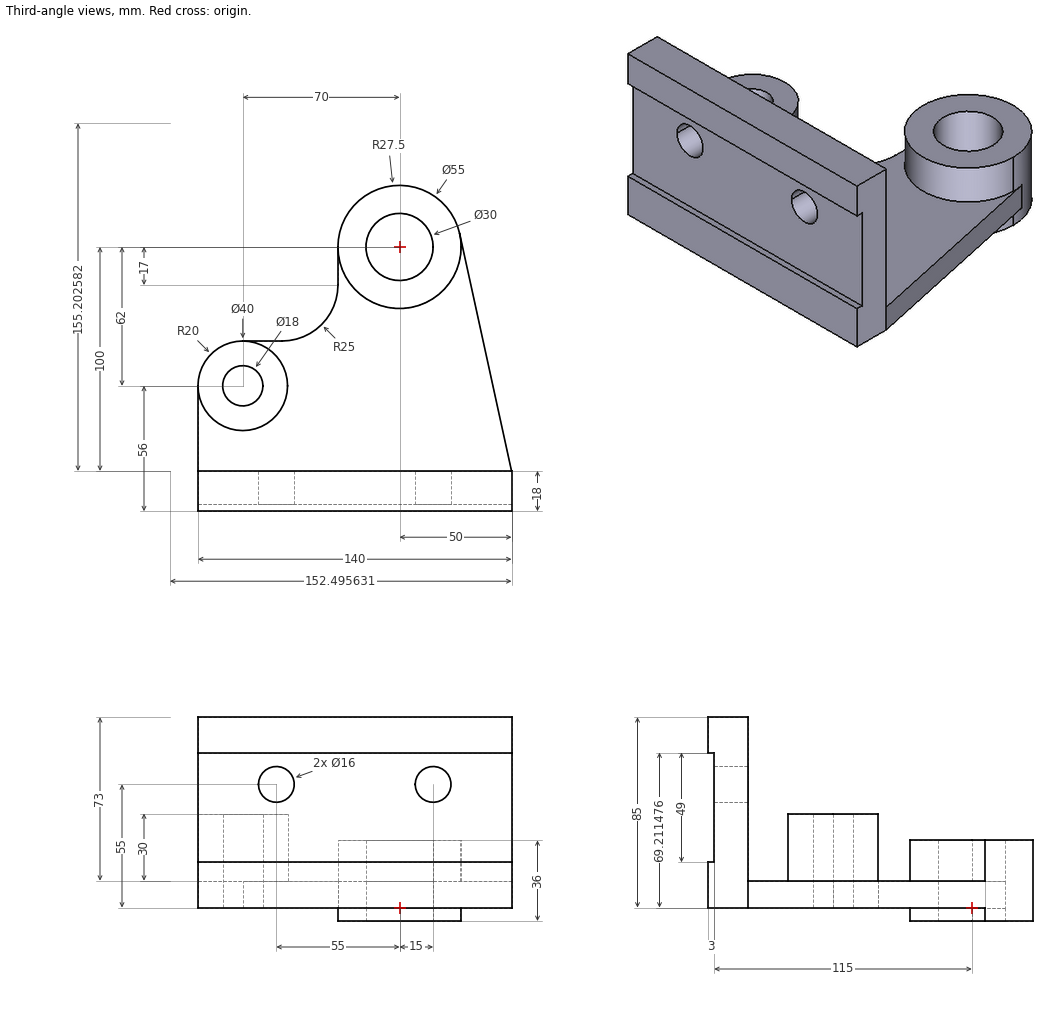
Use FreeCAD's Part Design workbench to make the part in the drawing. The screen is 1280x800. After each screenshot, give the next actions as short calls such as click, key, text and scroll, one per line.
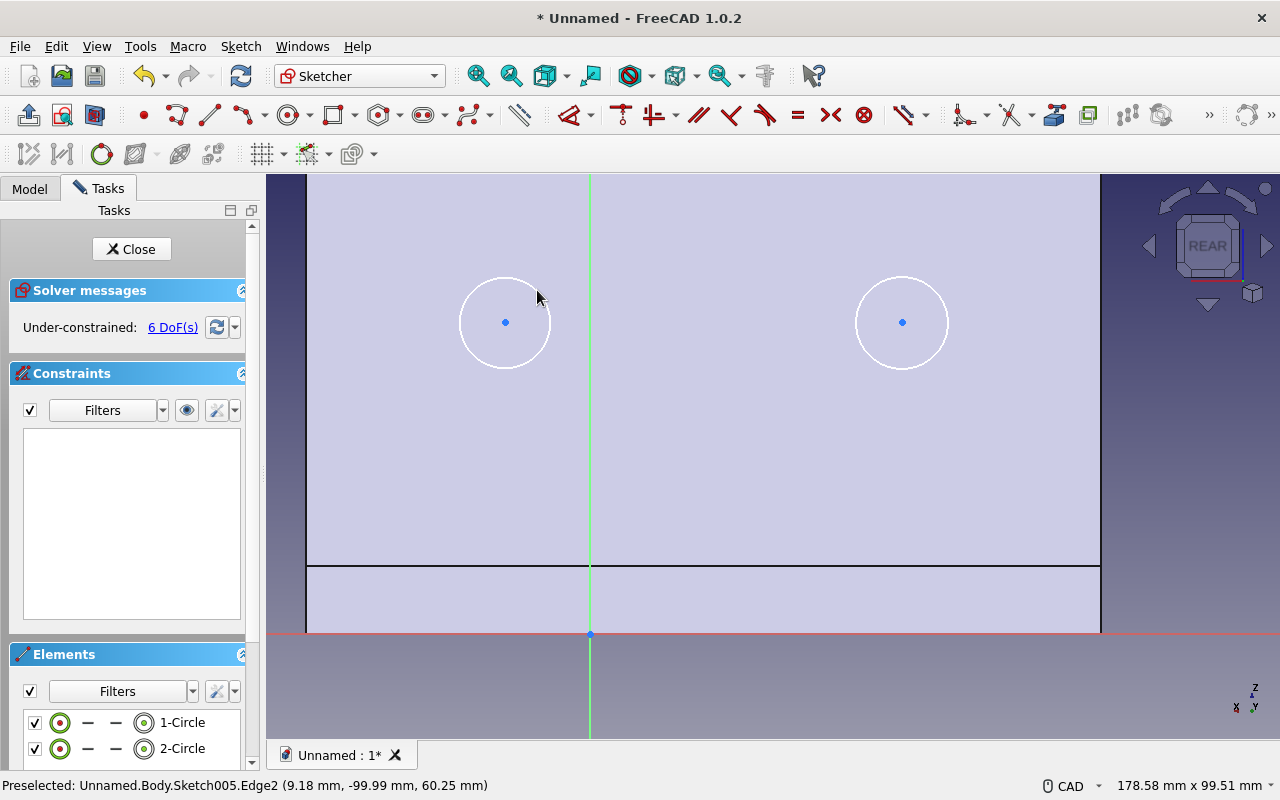
click(934, 290)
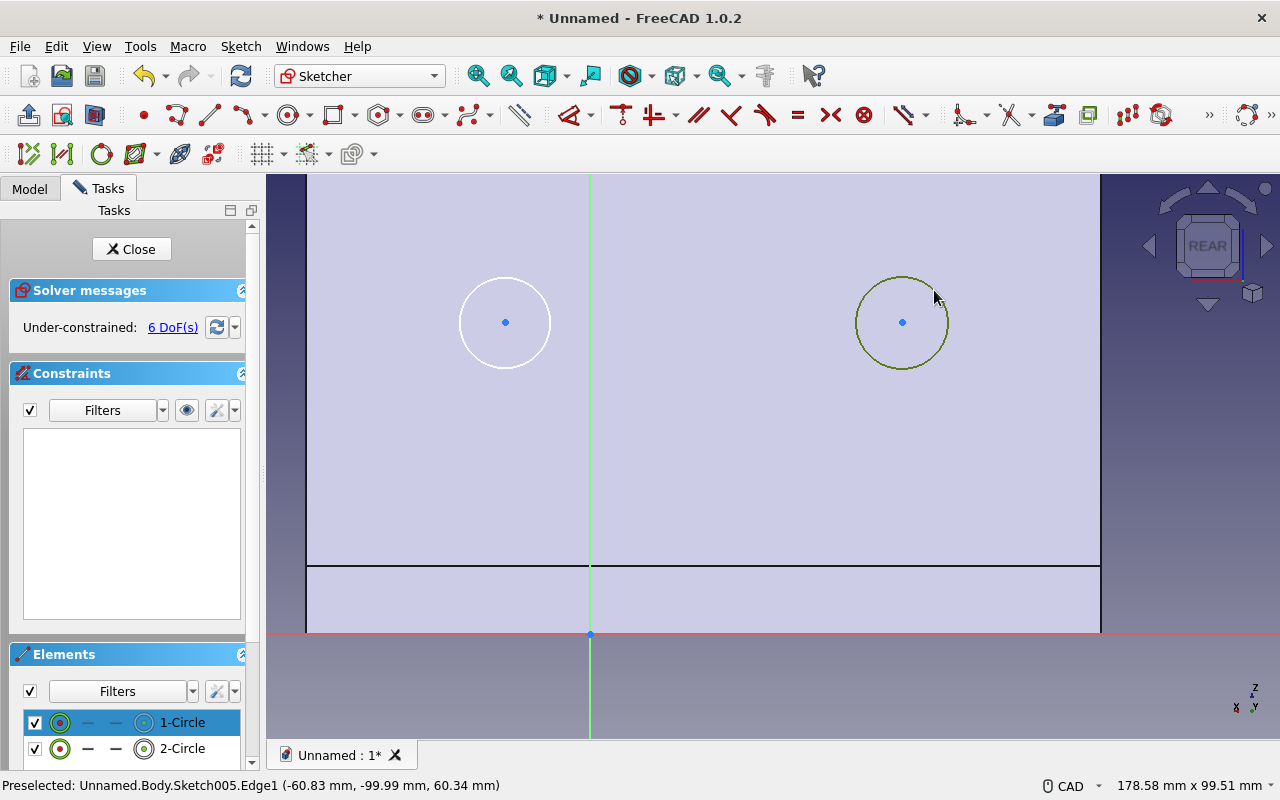
click(537, 291)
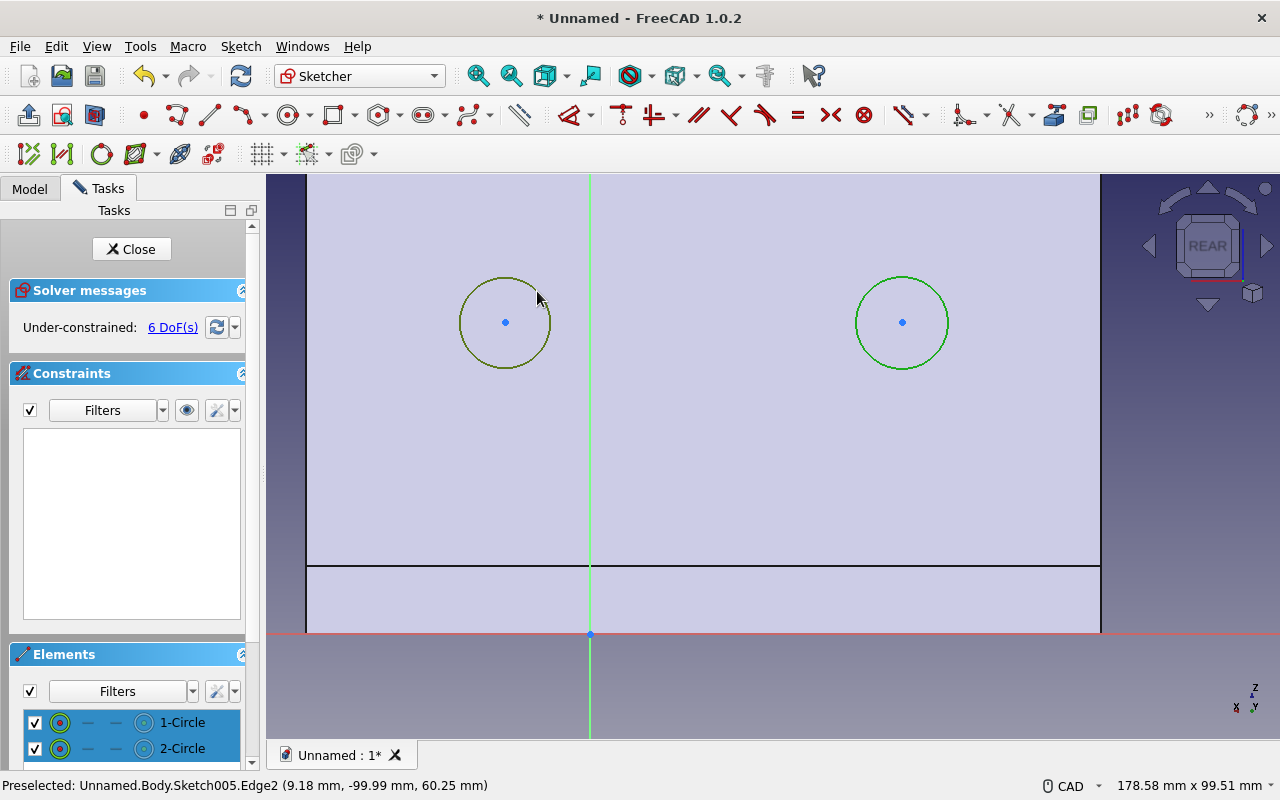
click(798, 116)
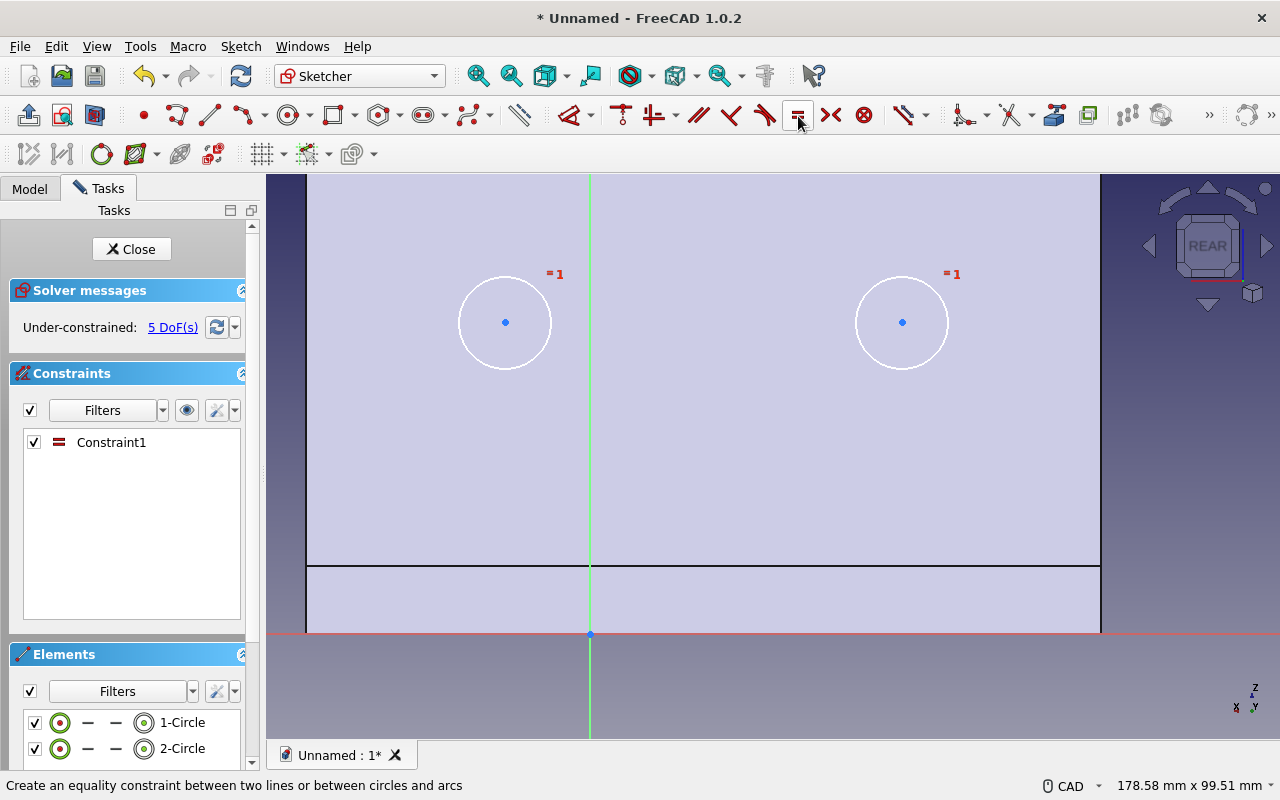
click(902, 323)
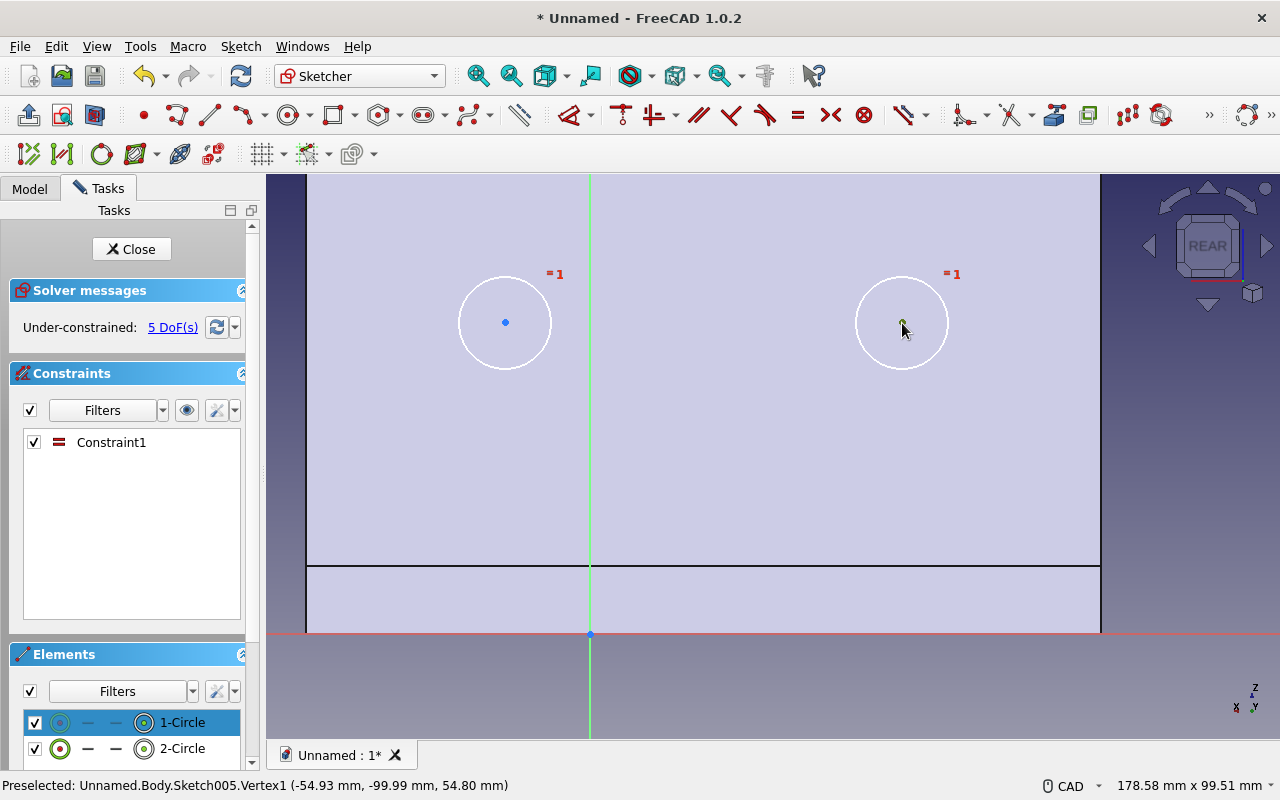
click(505, 323)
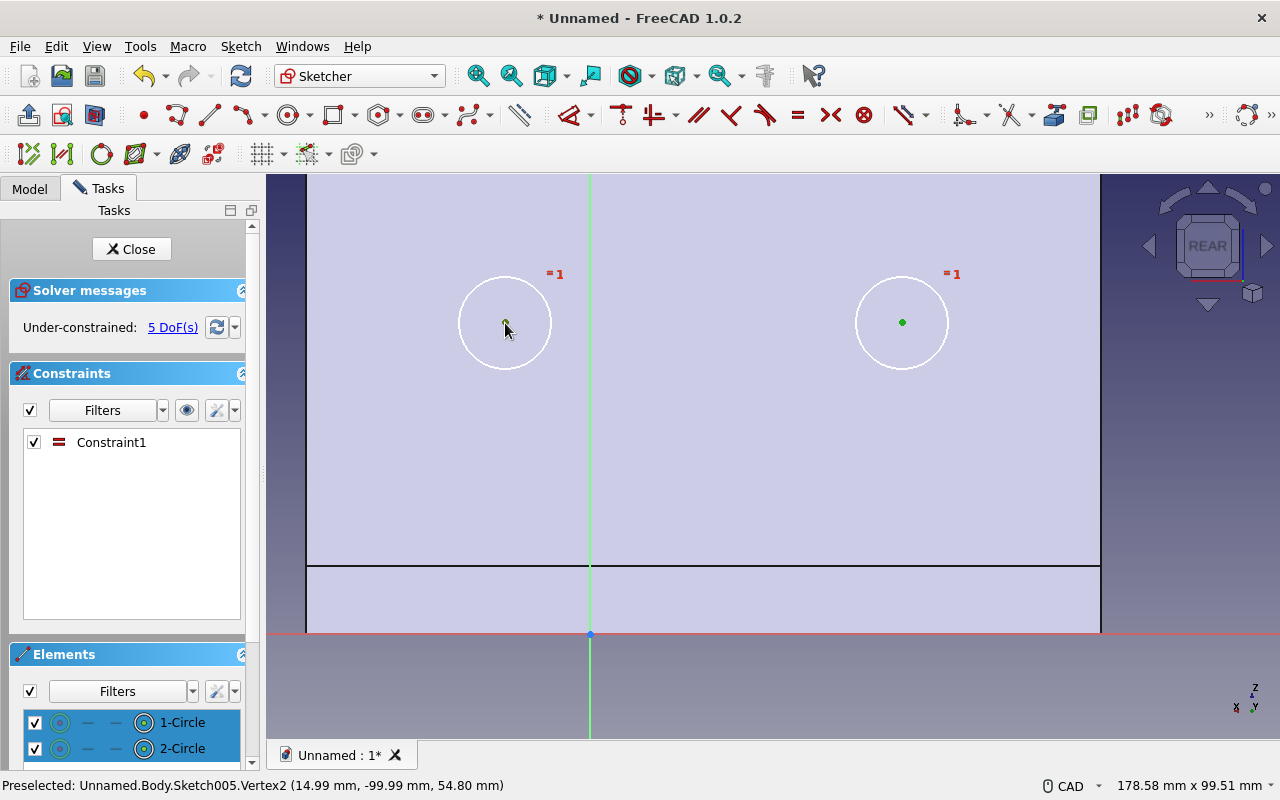
key(h)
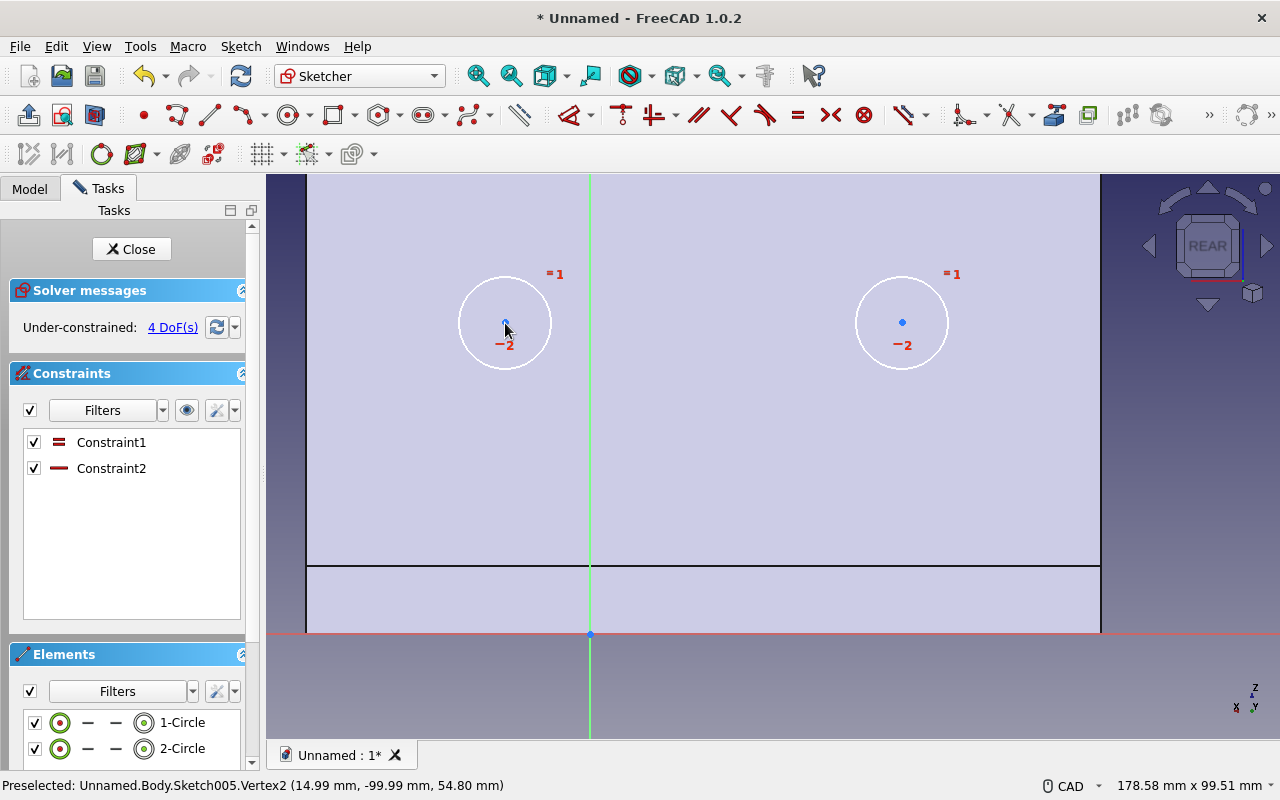
click(568, 116)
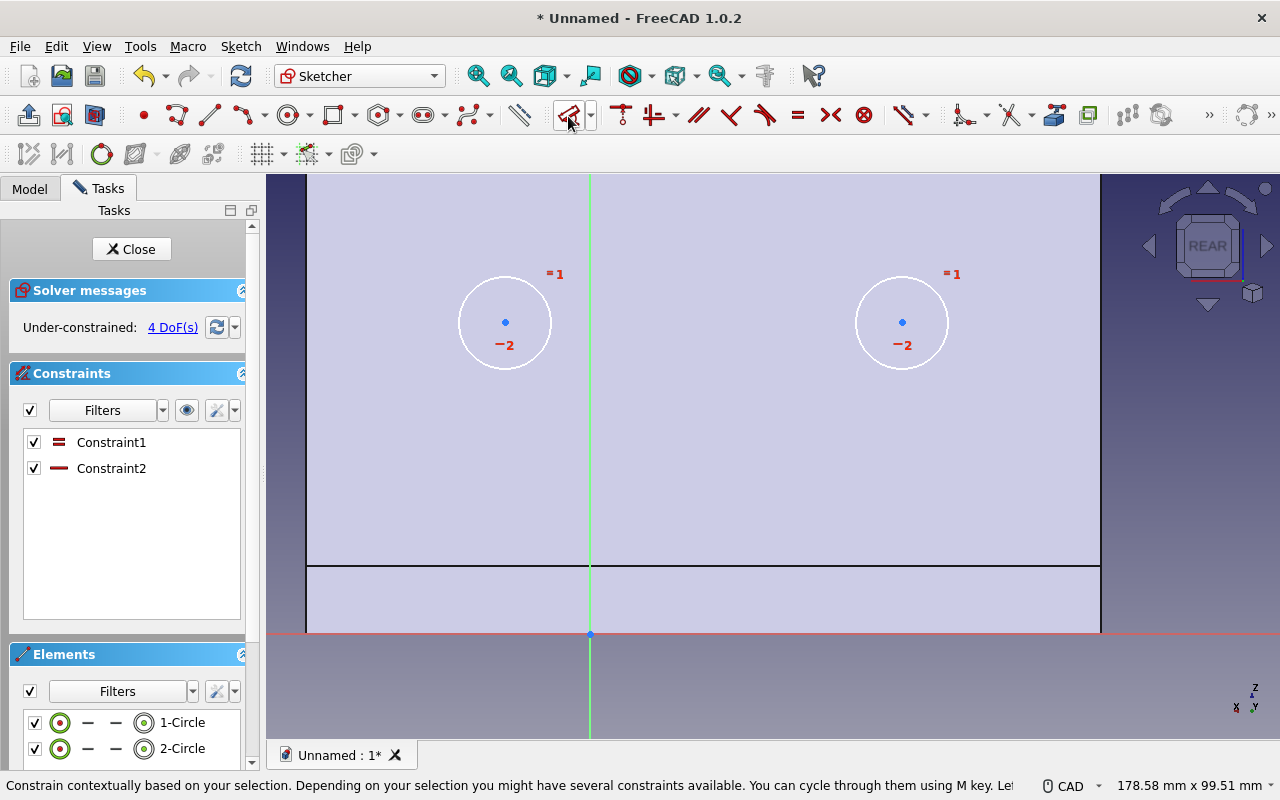
click(934, 290)
click(956, 267)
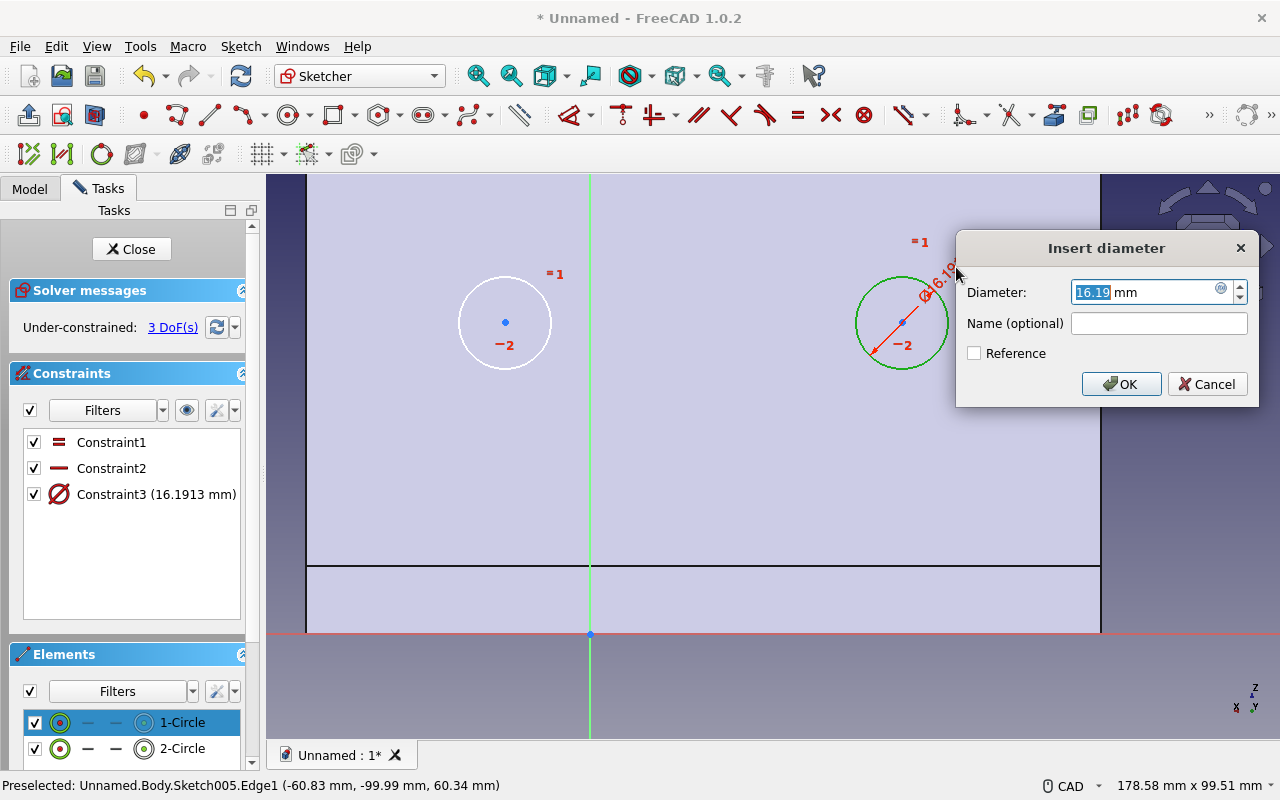
text(16)
key(Return)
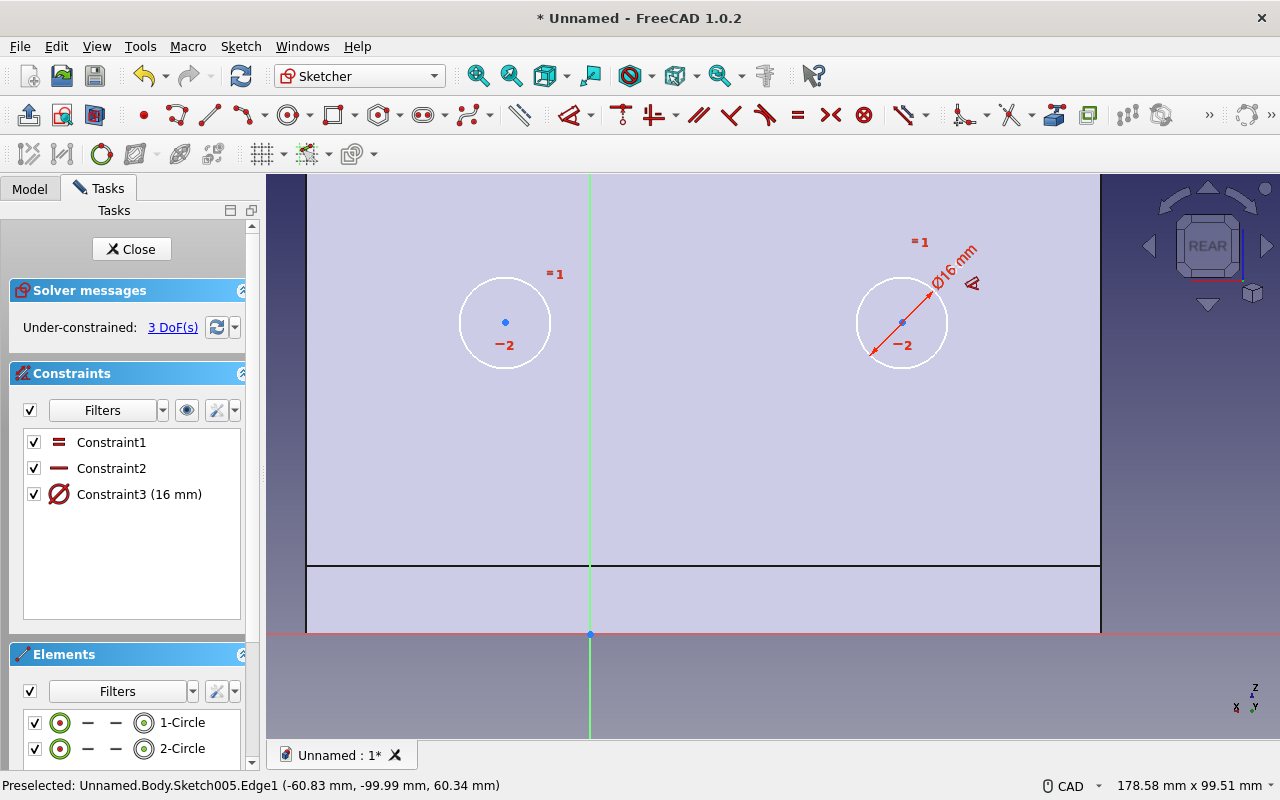
click(902, 323)
click(746, 668)